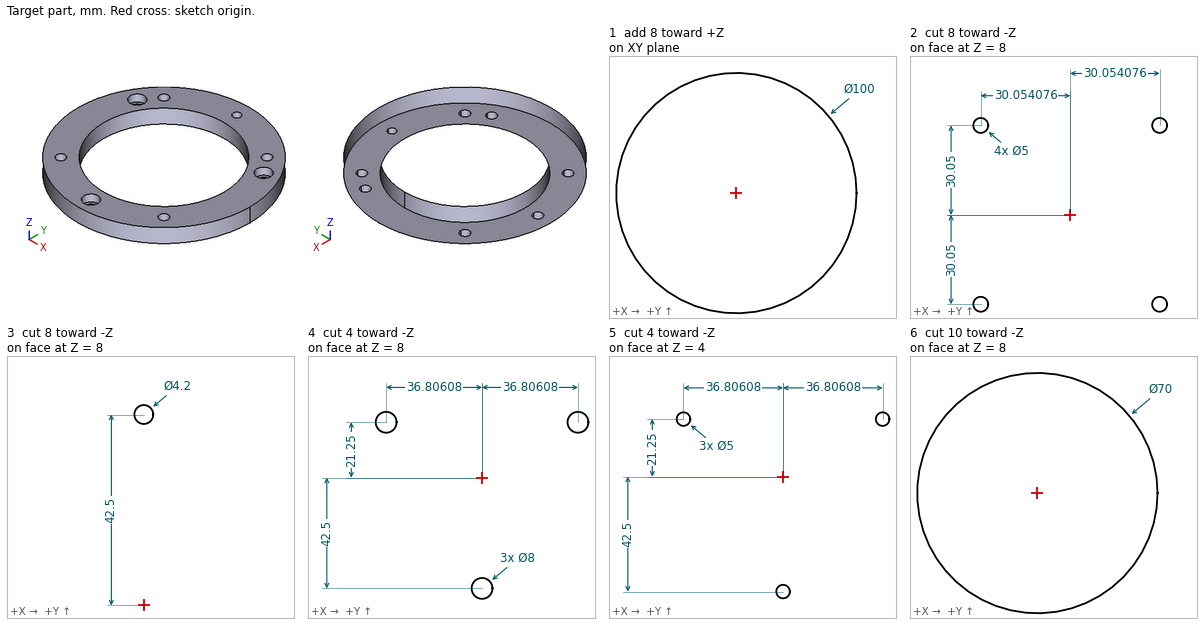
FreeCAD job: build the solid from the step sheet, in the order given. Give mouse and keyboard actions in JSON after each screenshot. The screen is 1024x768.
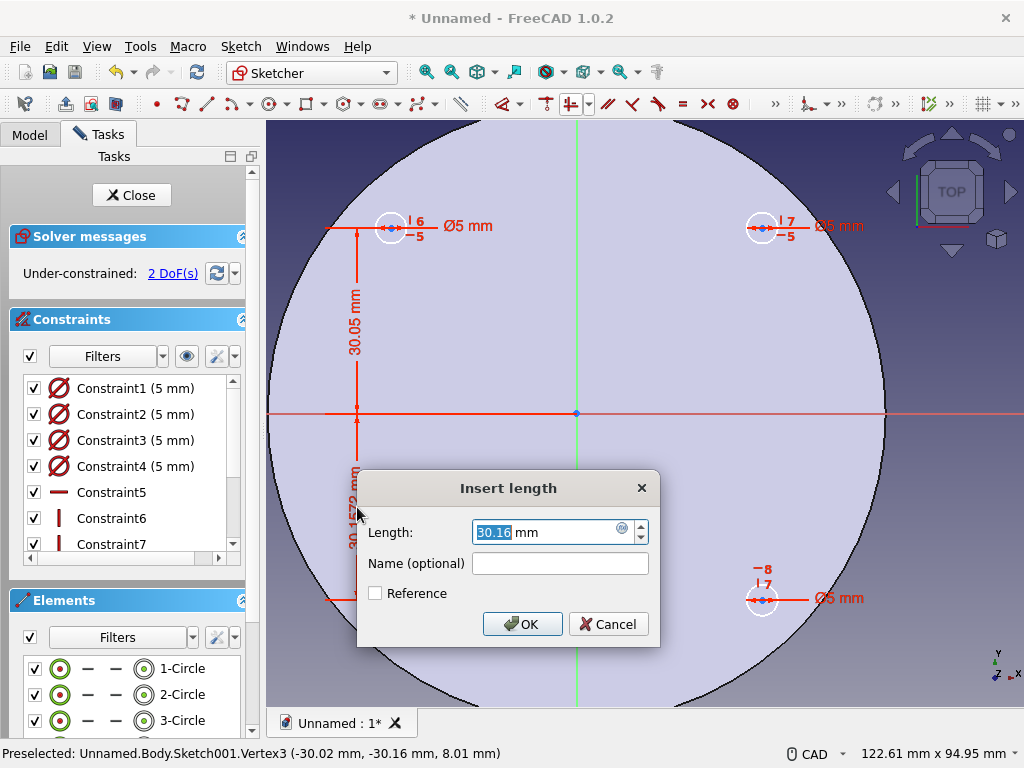
{"action": "type", "text": "30.05"}
{"action": "key", "text": "Return"}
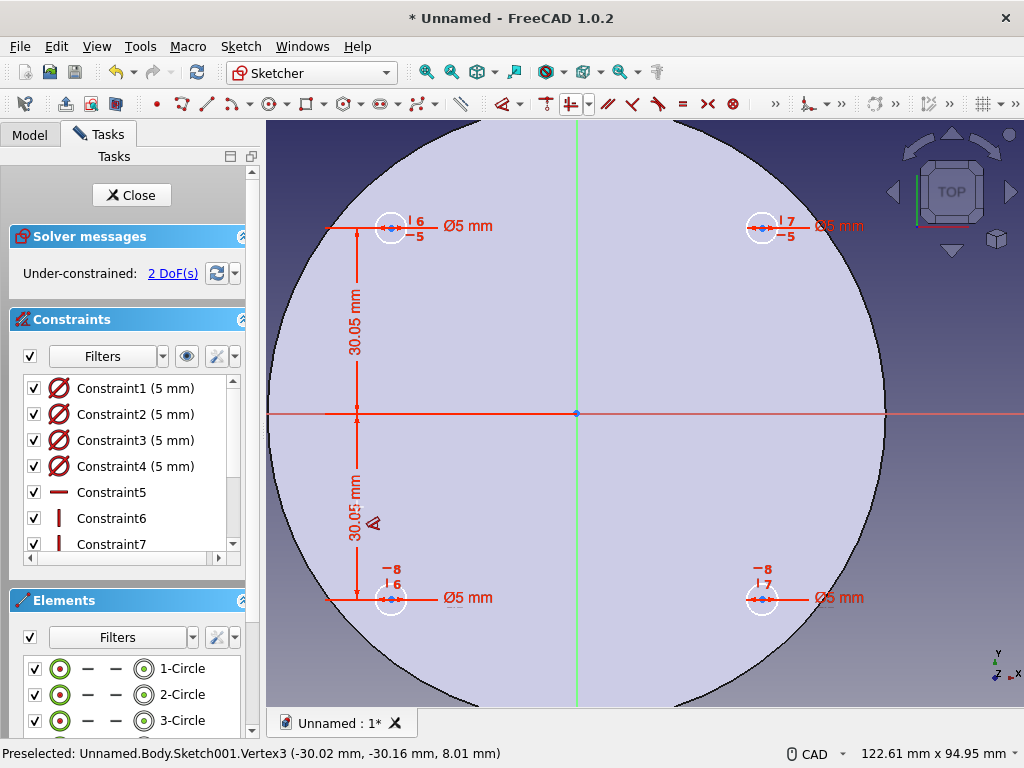
{"action": "left_click", "coordinate": [391, 228]}
{"action": "left_click", "coordinate": [484, 194]}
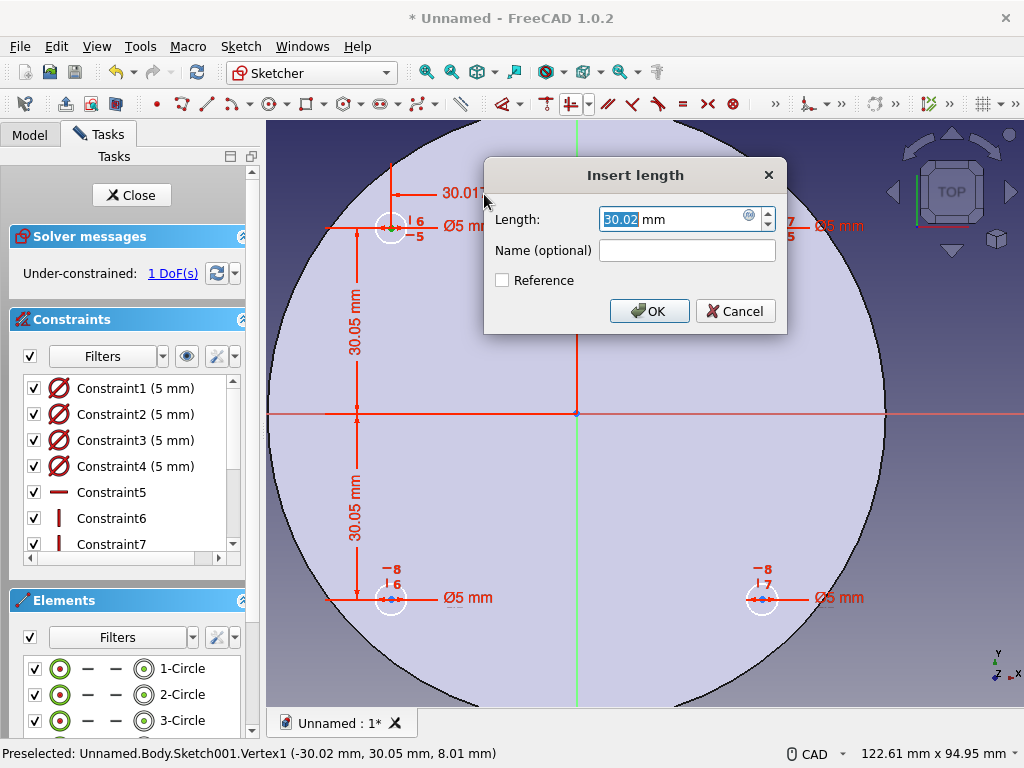
{"action": "type", "text": "30.054076"}
{"action": "key", "text": "Return"}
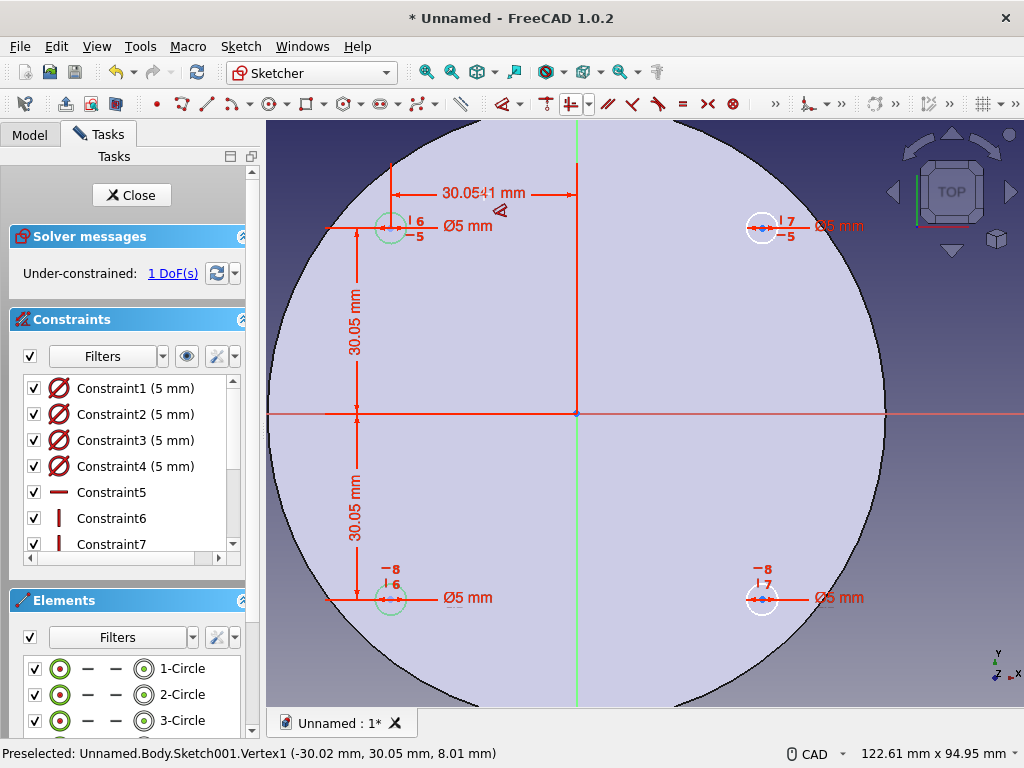
{"action": "left_click", "coordinate": [762, 228]}
{"action": "left_click", "coordinate": [669, 194]}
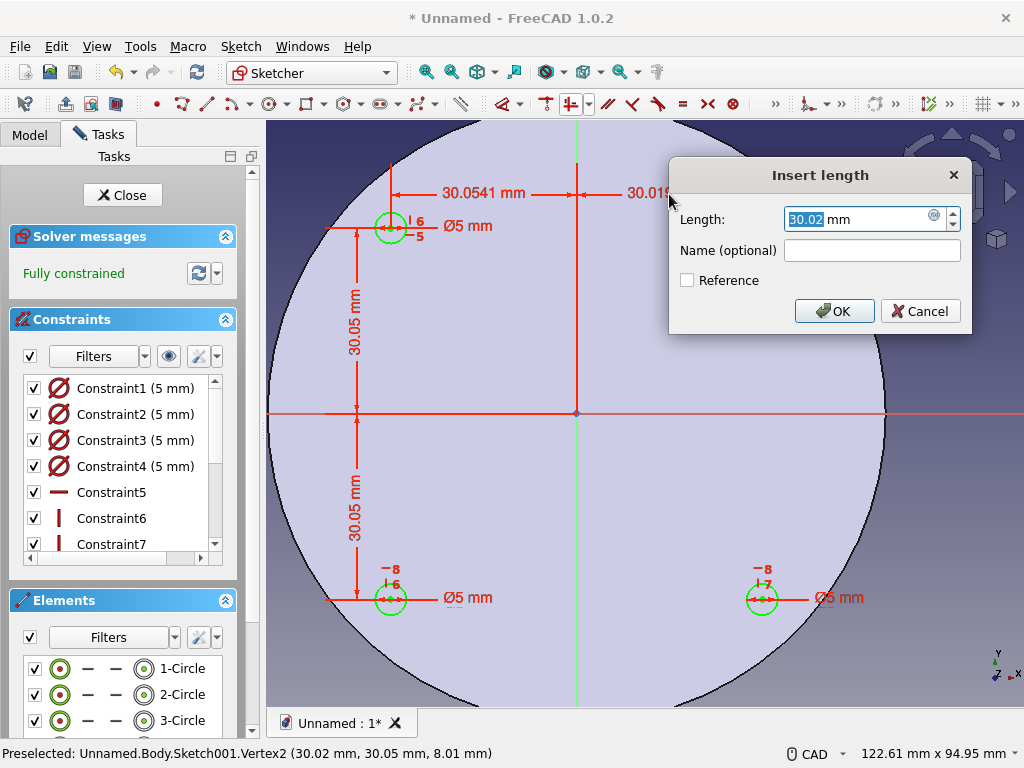
{"action": "type", "text": "30.054076"}
{"action": "key", "text": "Return"}
{"action": "key", "text": "Escape"}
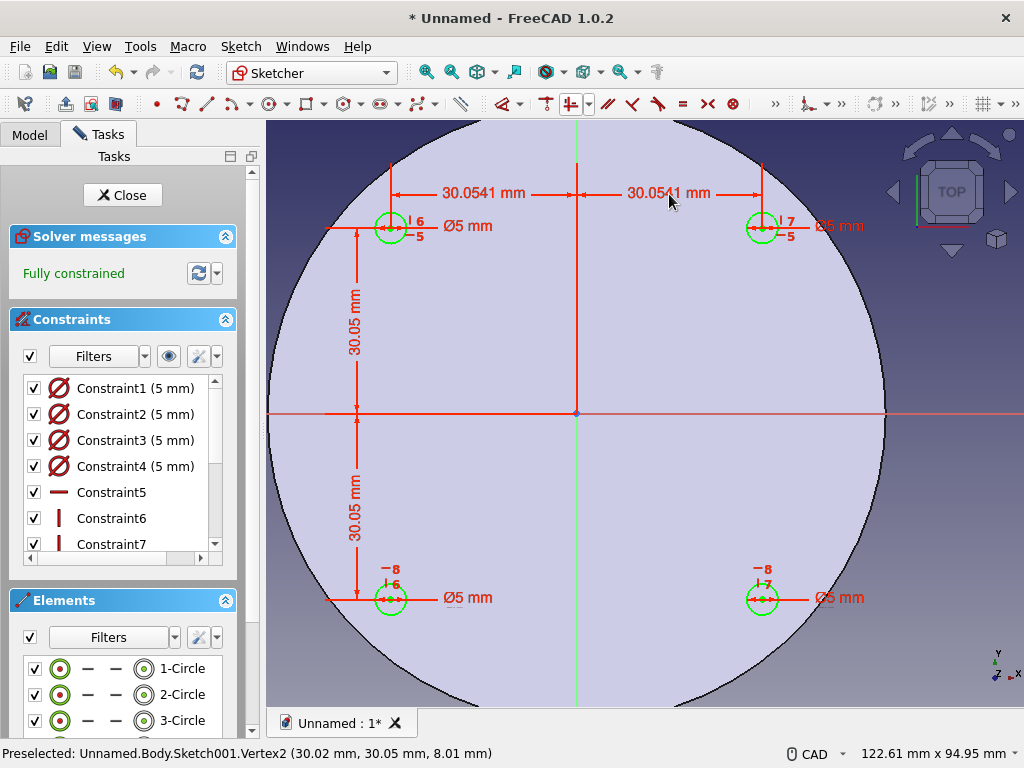
{"action": "left_click", "coordinate": [123, 195]}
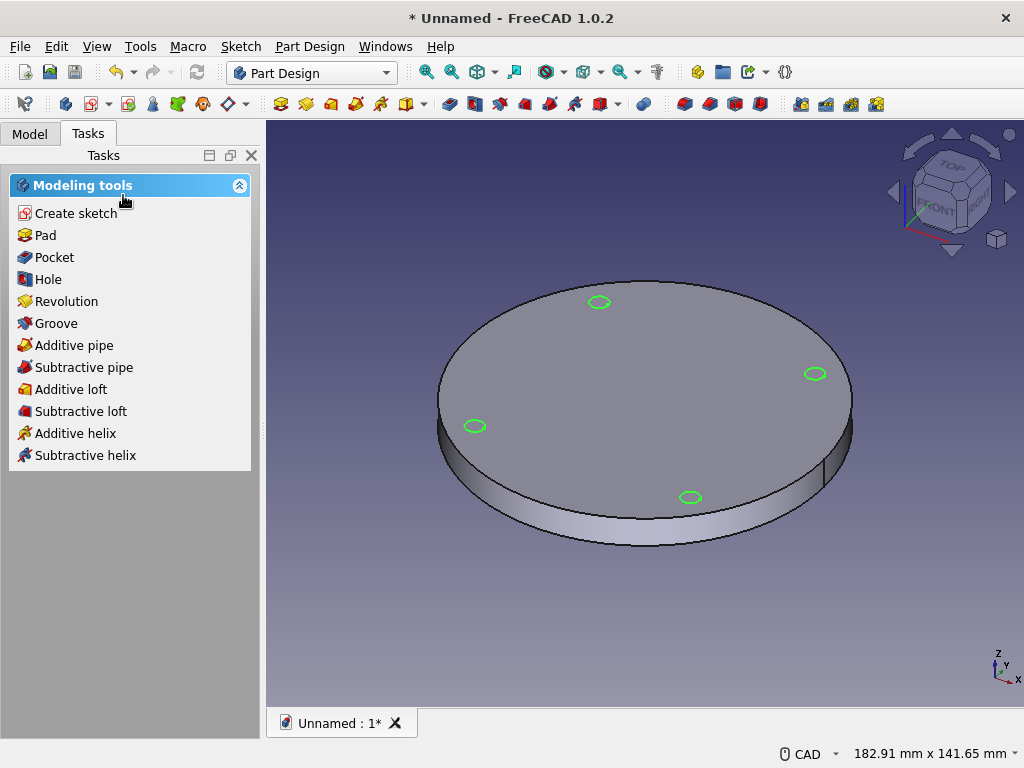
{"action": "left_click", "coordinate": [450, 104]}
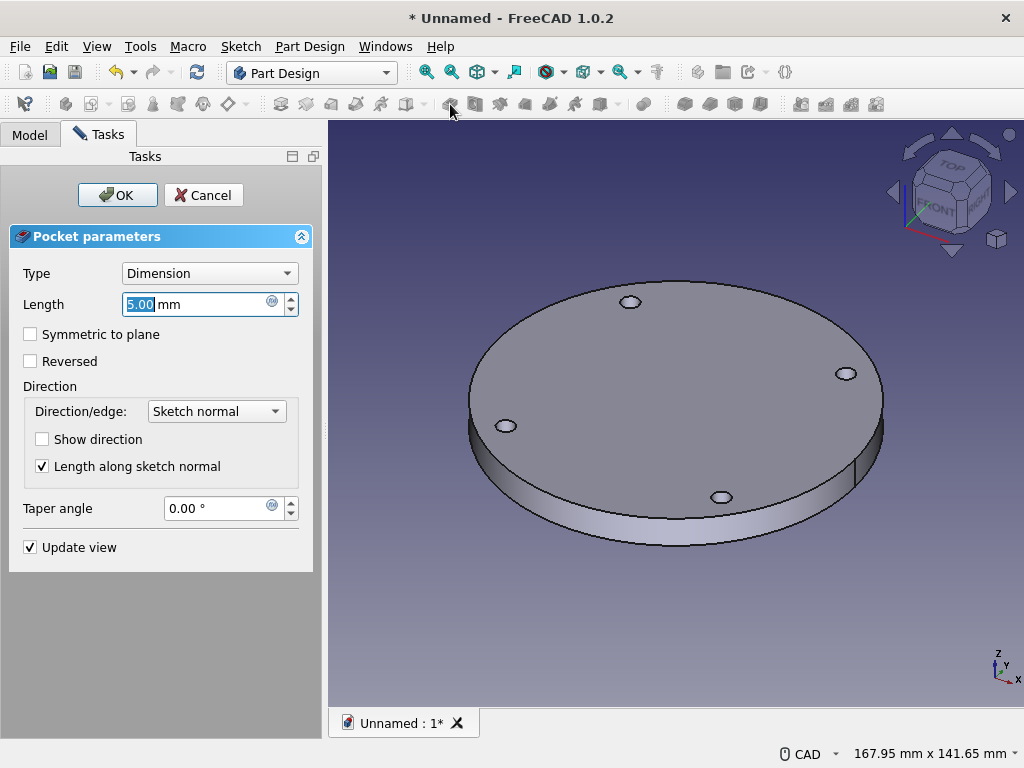
{"action": "type", "text": "8"}
{"action": "key", "text": "Tab"}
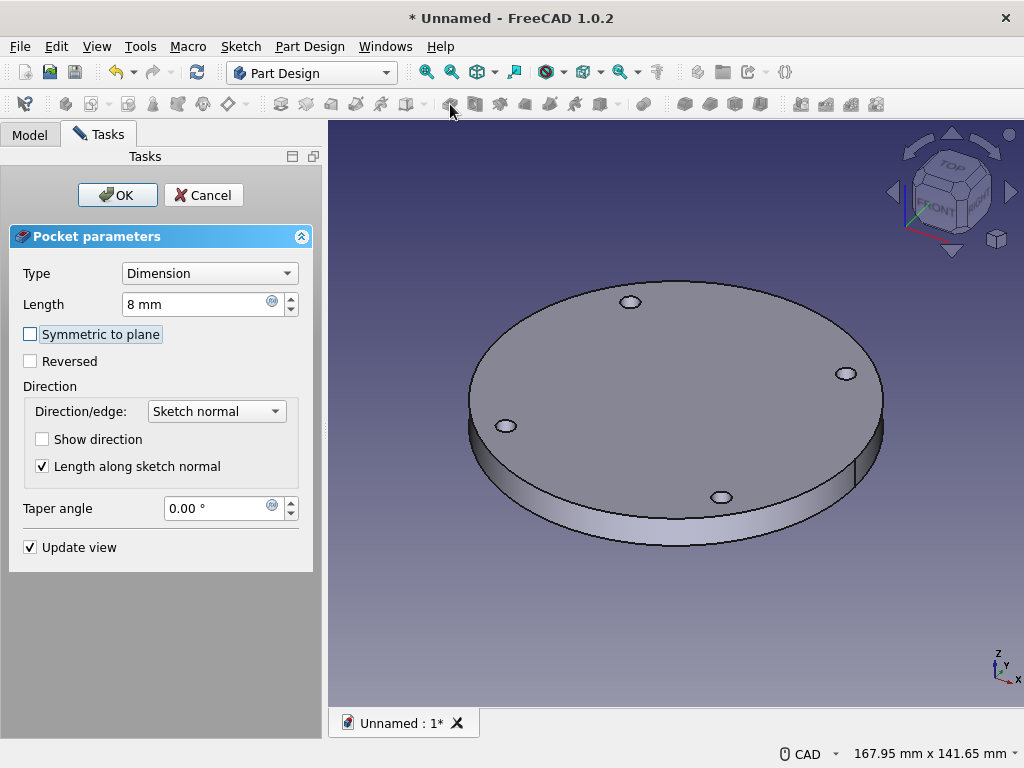
{"action": "left_click", "coordinate": [118, 195]}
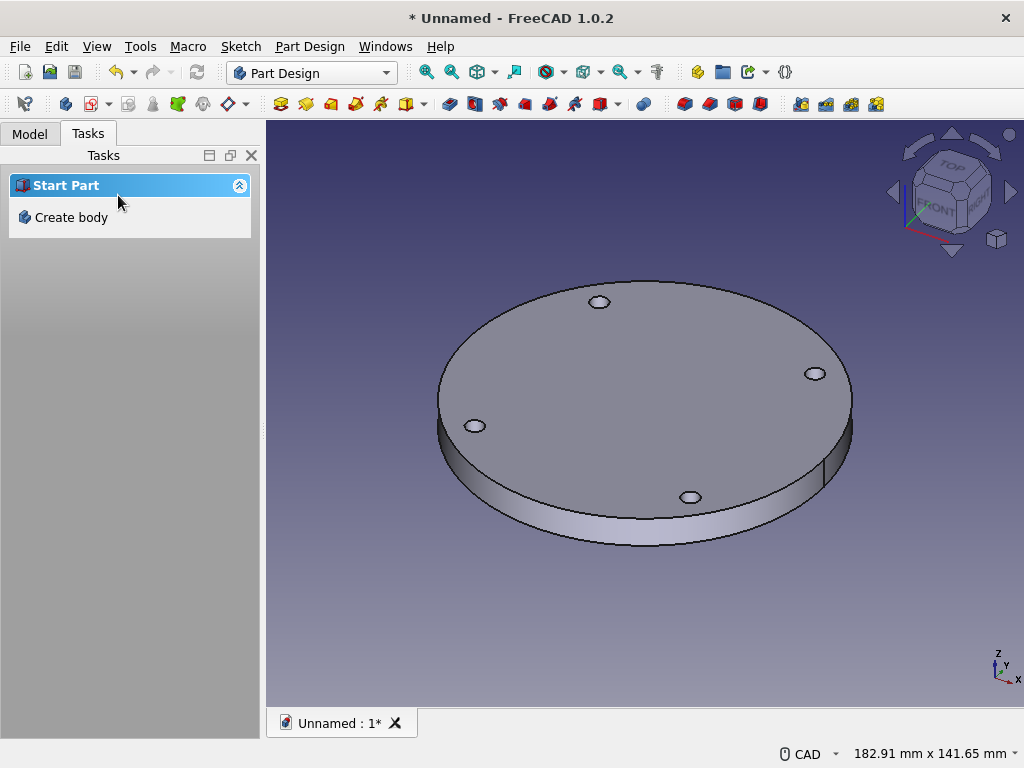
{"action": "left_click", "coordinate": [645, 399]}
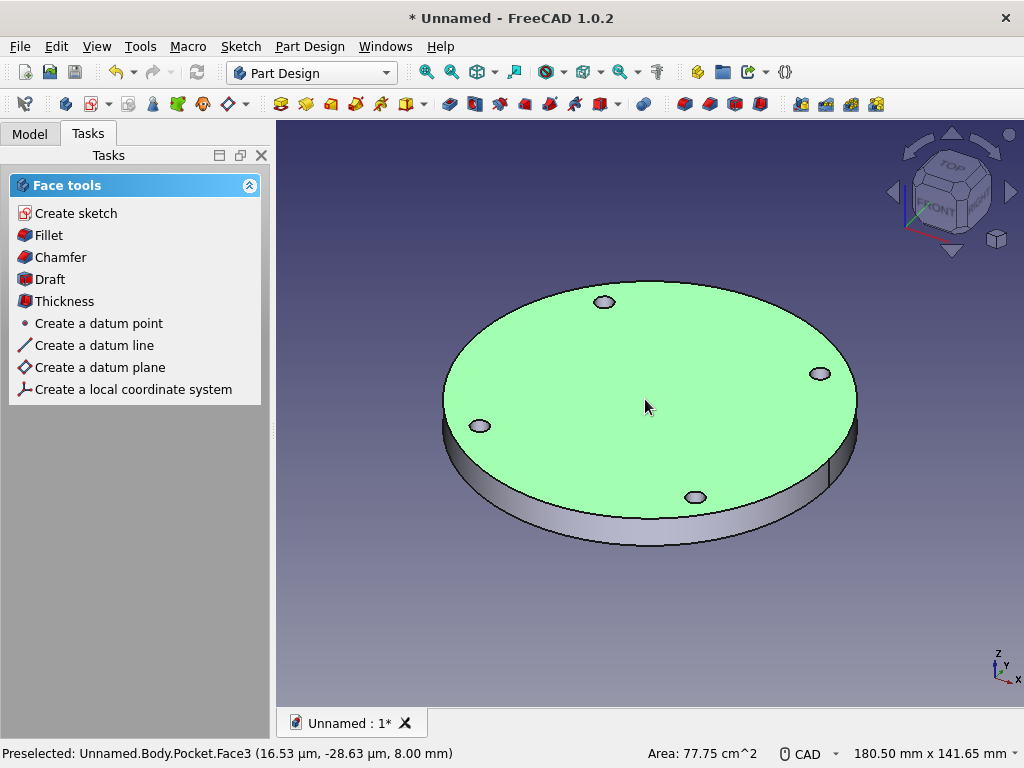
{"action": "left_click", "coordinate": [90, 104]}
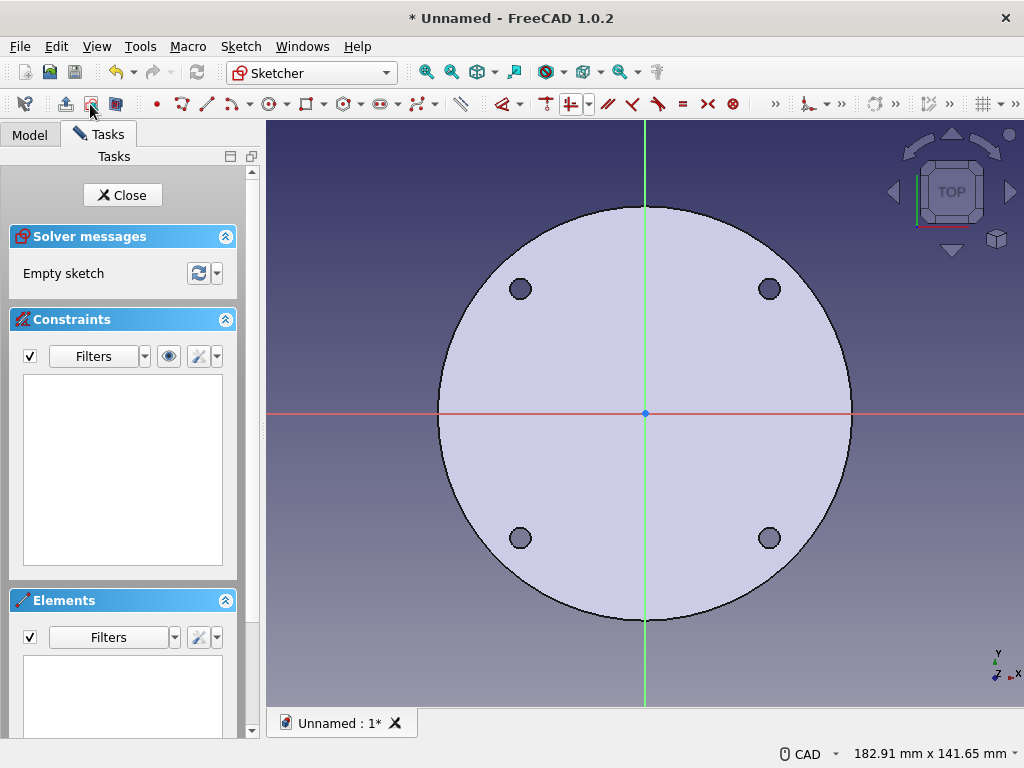
{"action": "scroll", "coordinate": [649, 228], "scroll_direction": "up", "scroll_amount": 15}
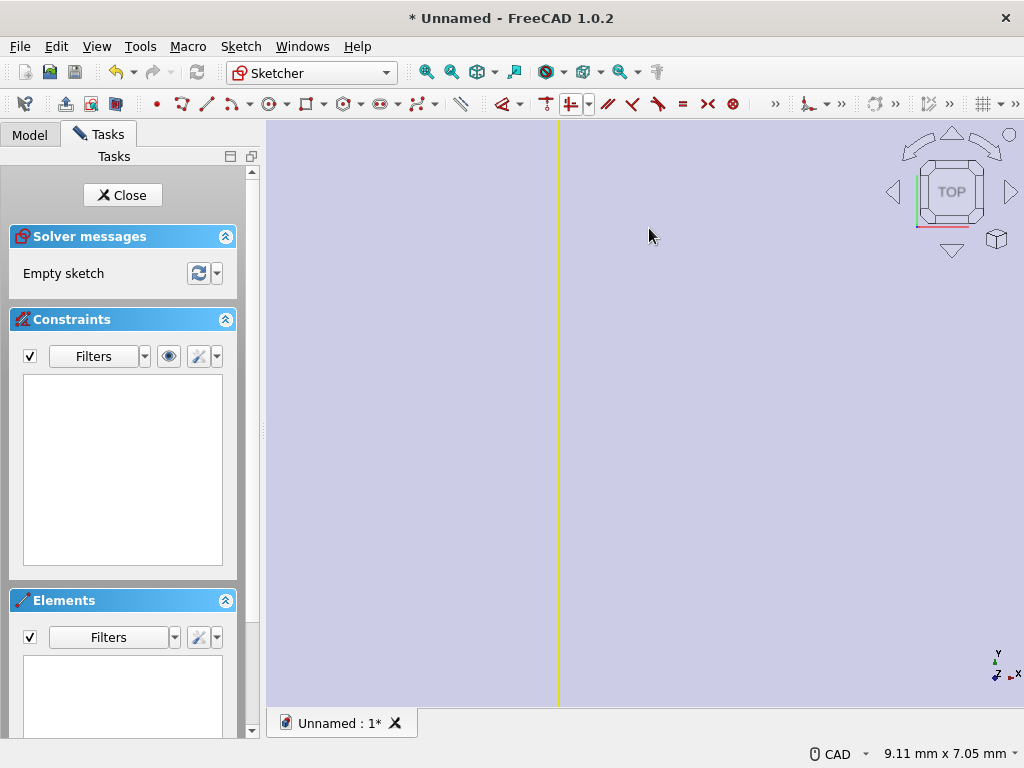
{"action": "left_click", "coordinate": [268, 104]}